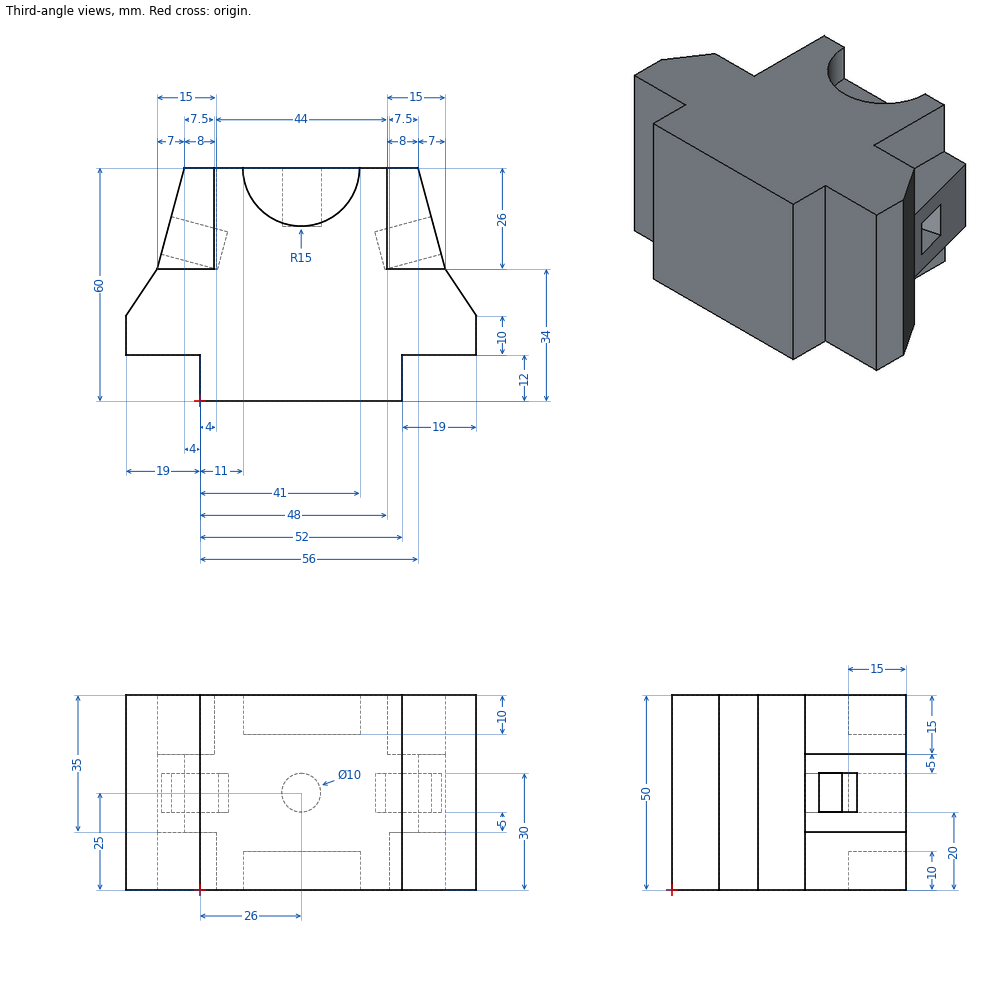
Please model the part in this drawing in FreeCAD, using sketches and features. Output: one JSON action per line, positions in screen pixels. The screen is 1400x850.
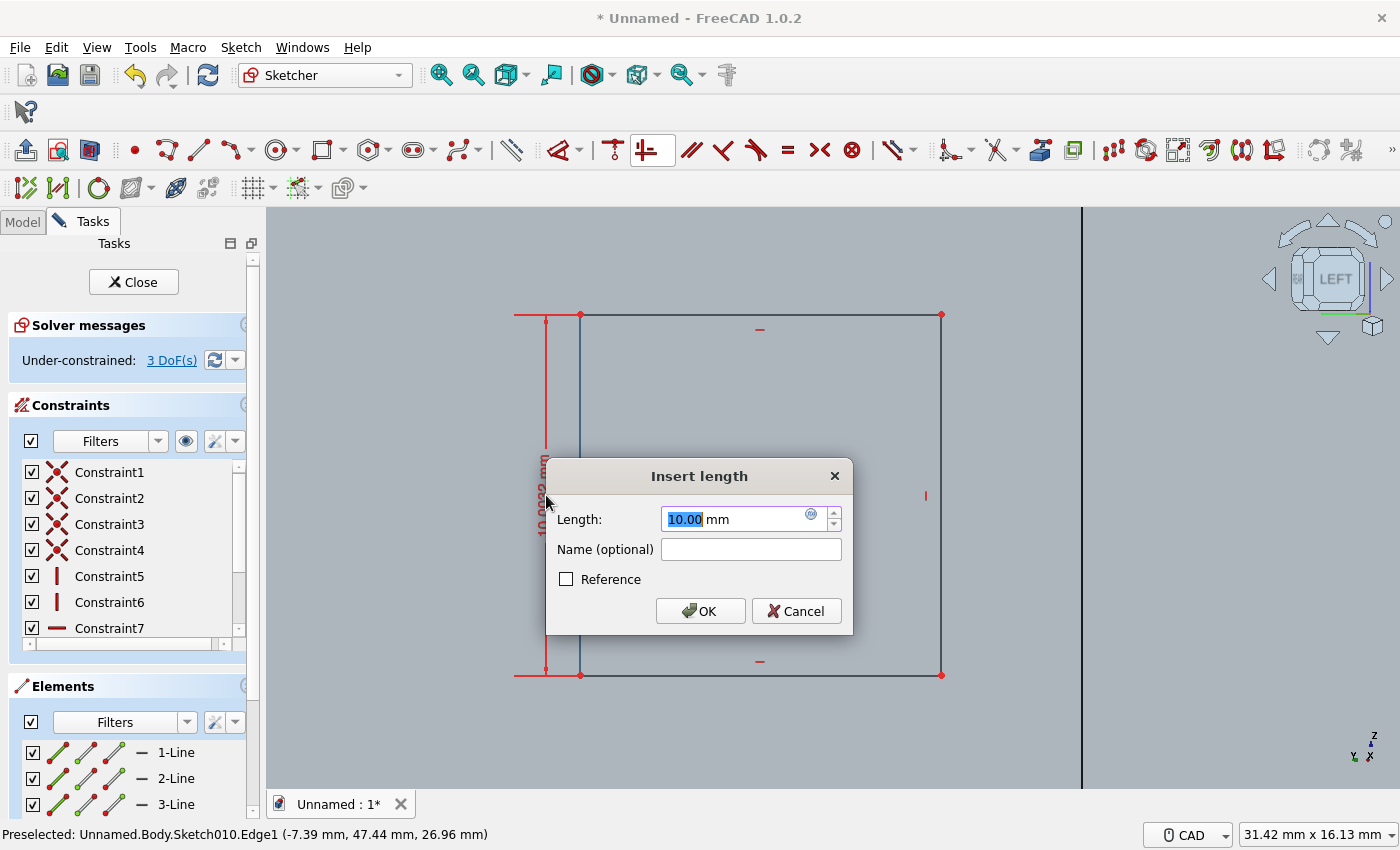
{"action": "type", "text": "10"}
{"action": "key", "text": "Return"}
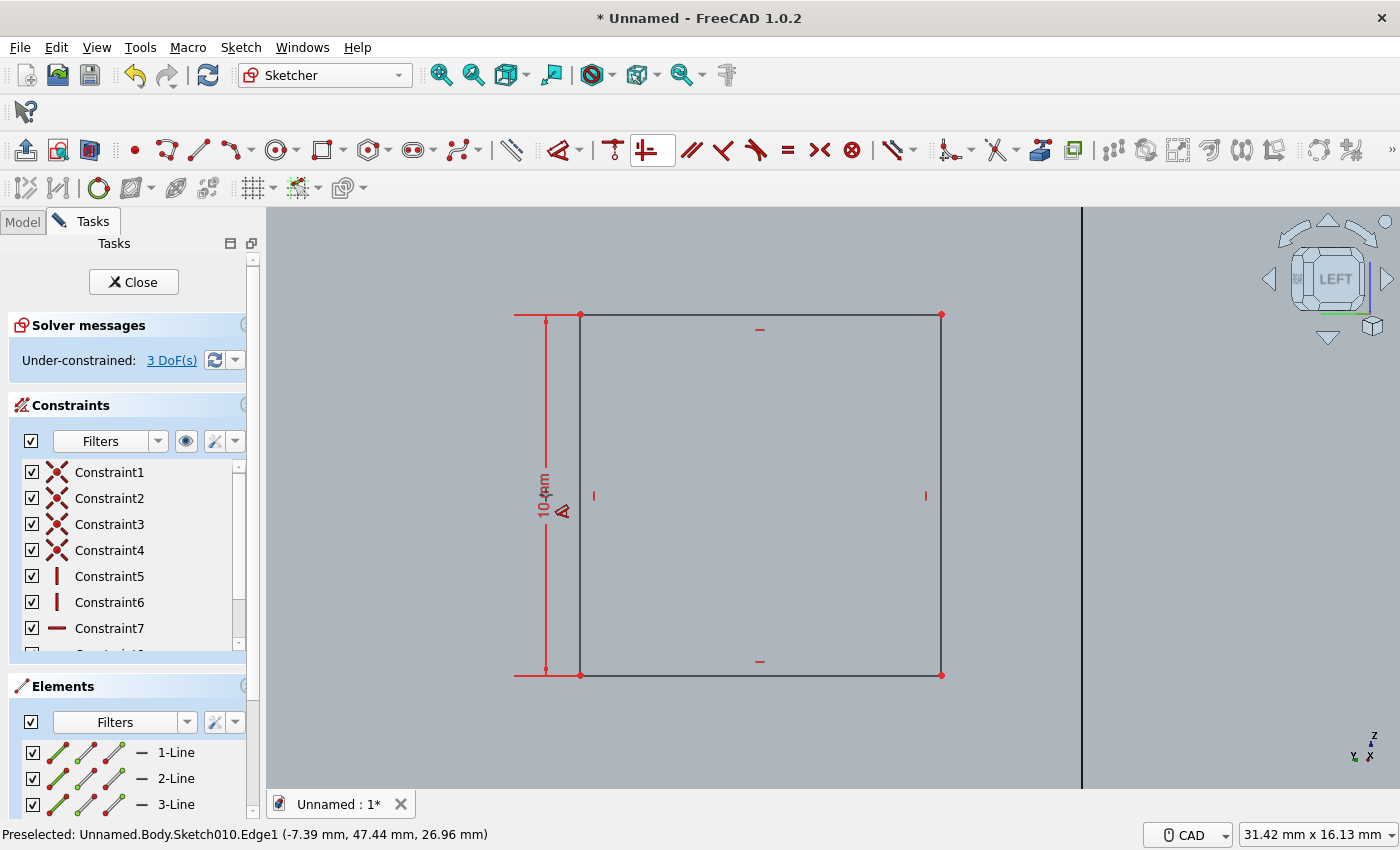
{"action": "left_click", "coordinate": [688, 676]}
{"action": "left_click", "coordinate": [760, 710]}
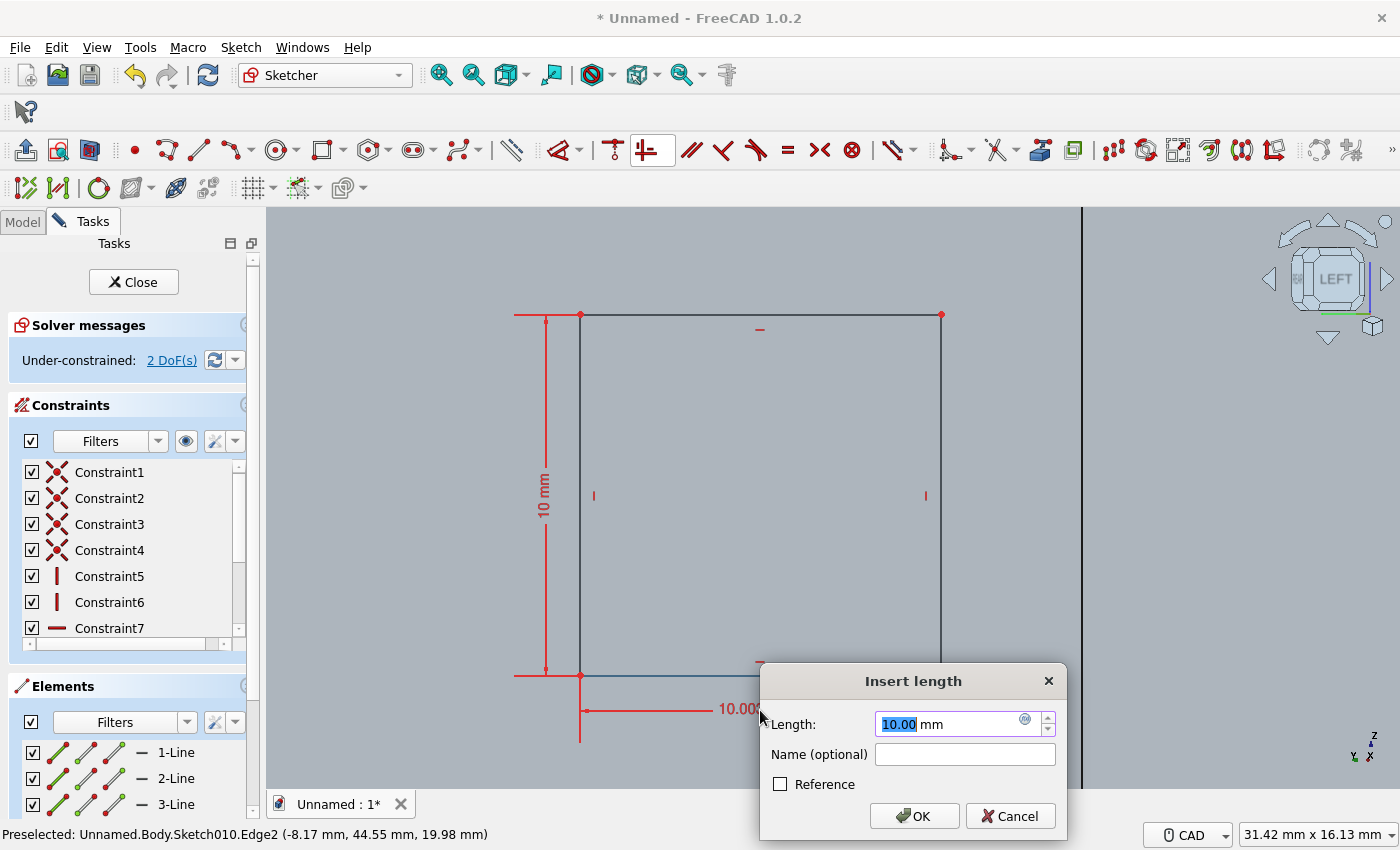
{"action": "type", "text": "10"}
{"action": "key", "text": "Return"}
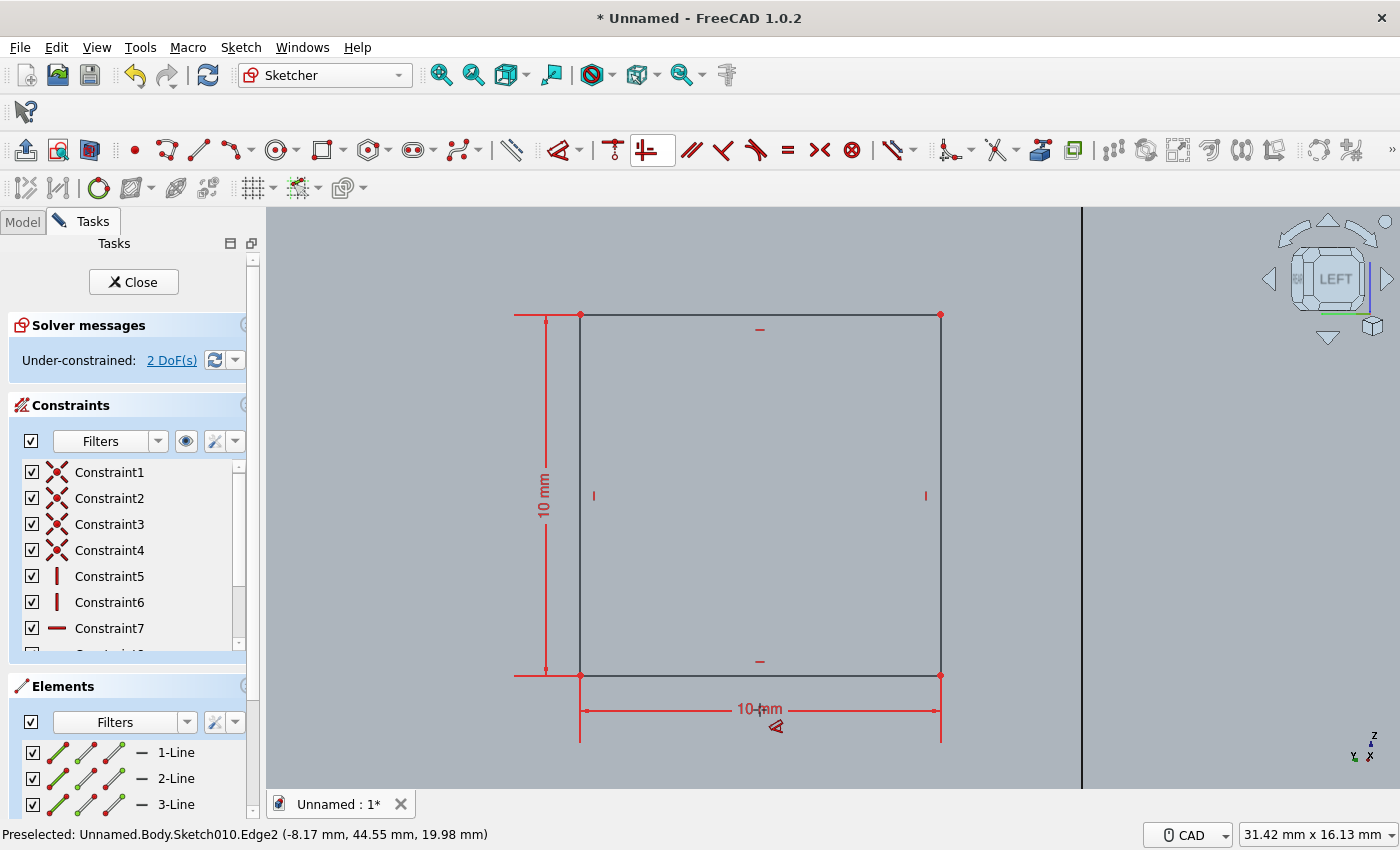
{"action": "left_click", "coordinate": [580, 315]}
{"action": "left_click", "coordinate": [546, 538]}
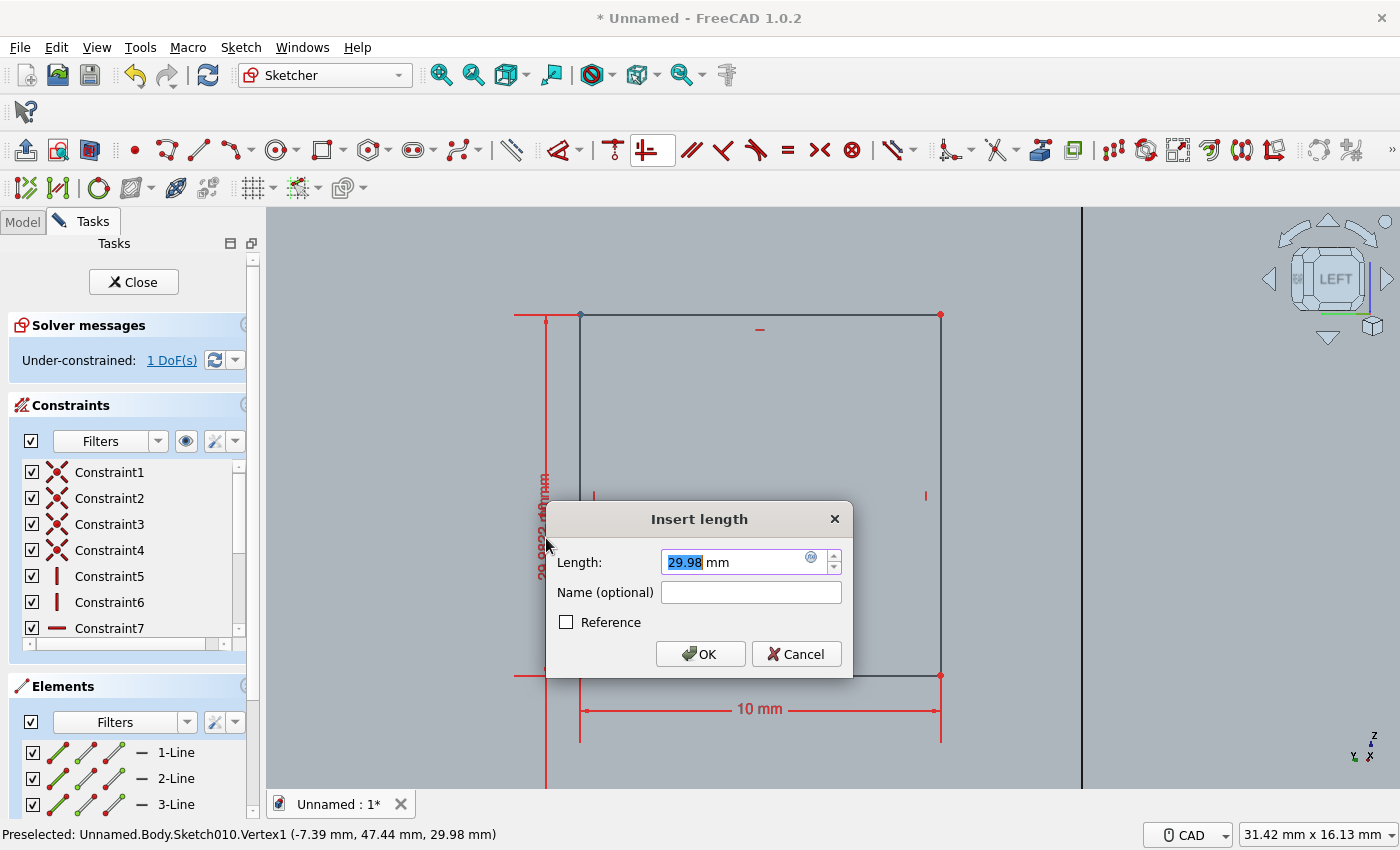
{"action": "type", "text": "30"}
{"action": "key", "text": "Return"}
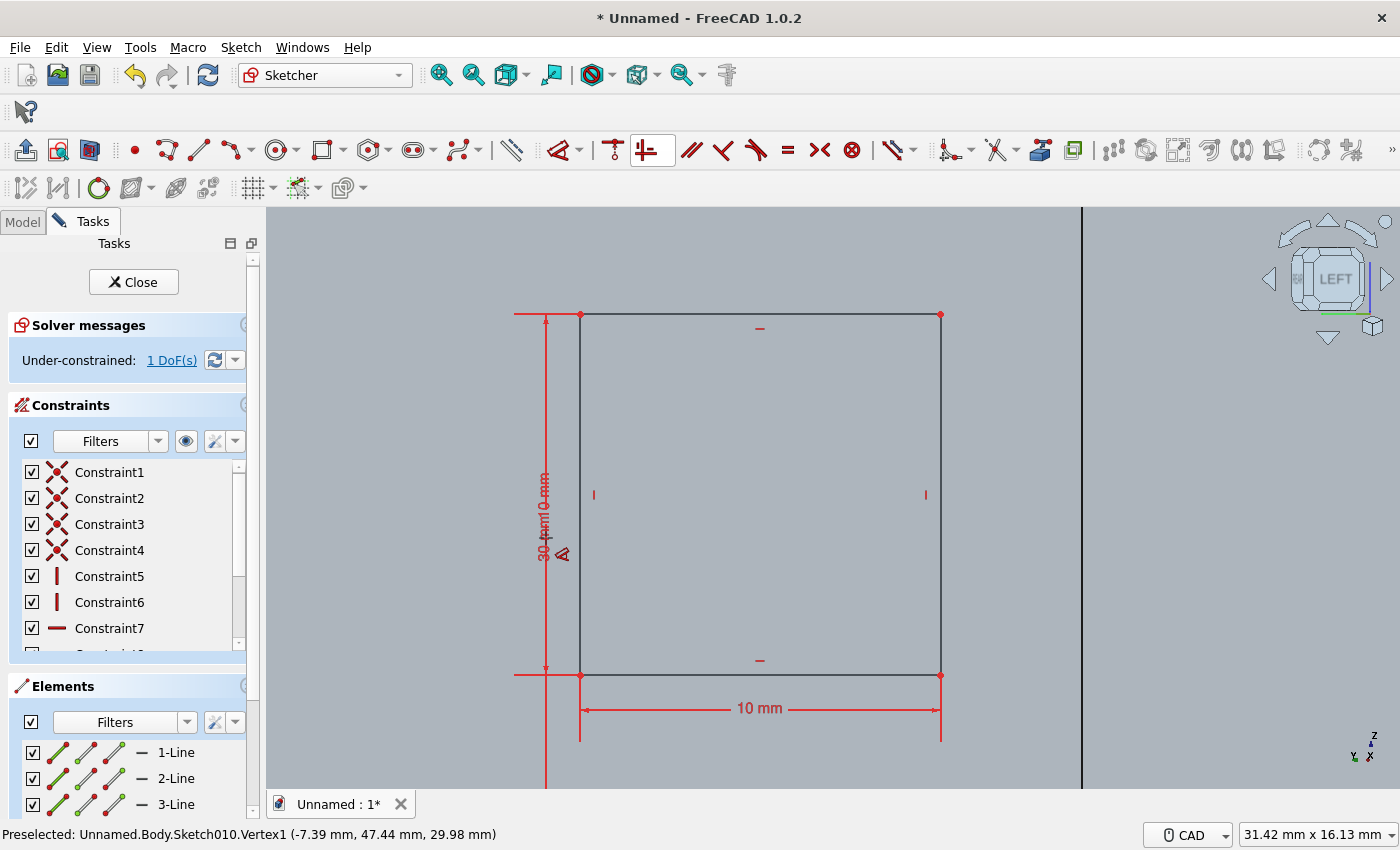
{"action": "left_click", "coordinate": [580, 314]}
{"action": "left_click", "coordinate": [907, 280]}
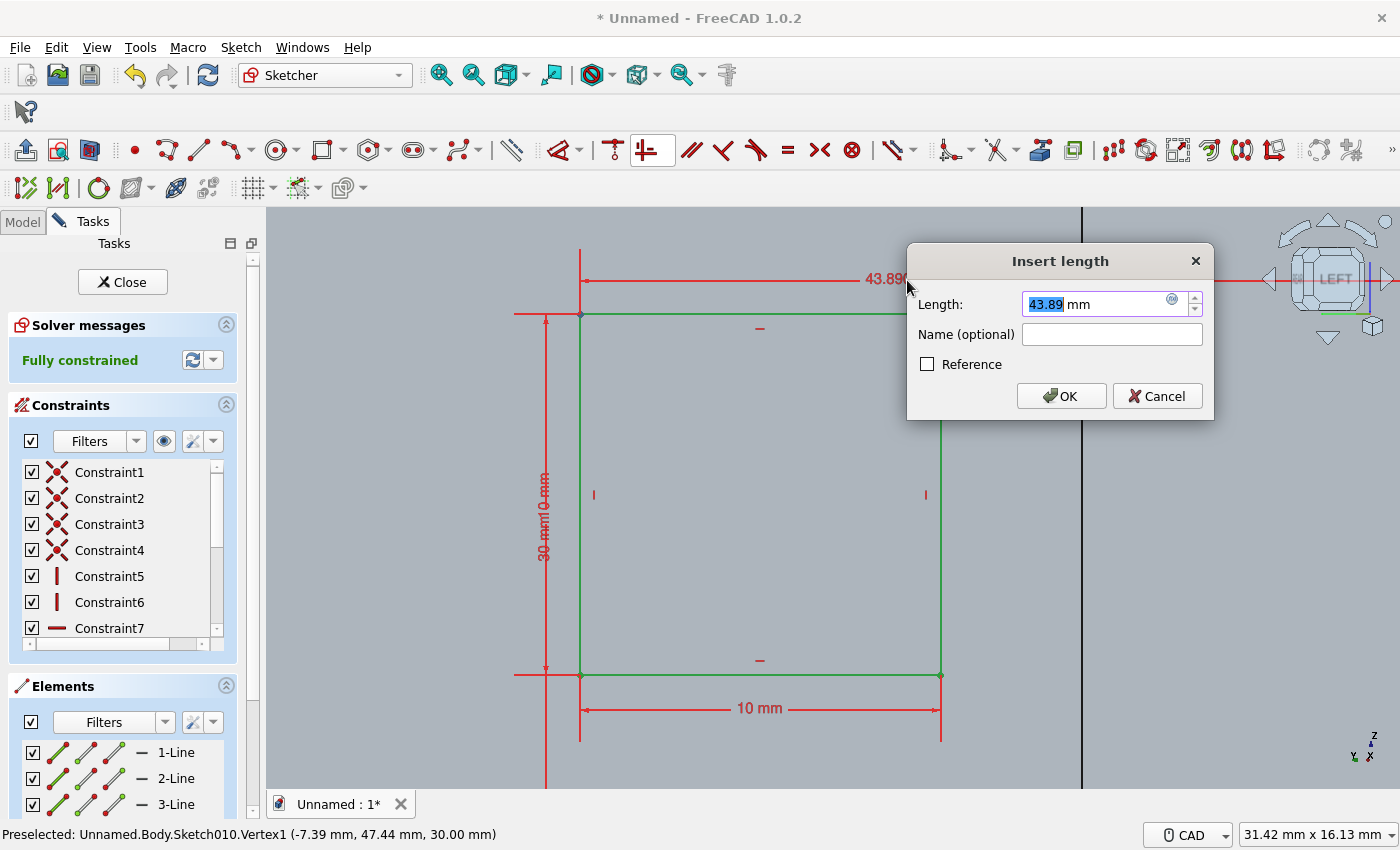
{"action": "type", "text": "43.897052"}
{"action": "key", "text": "Return"}
{"action": "key", "text": "Escape"}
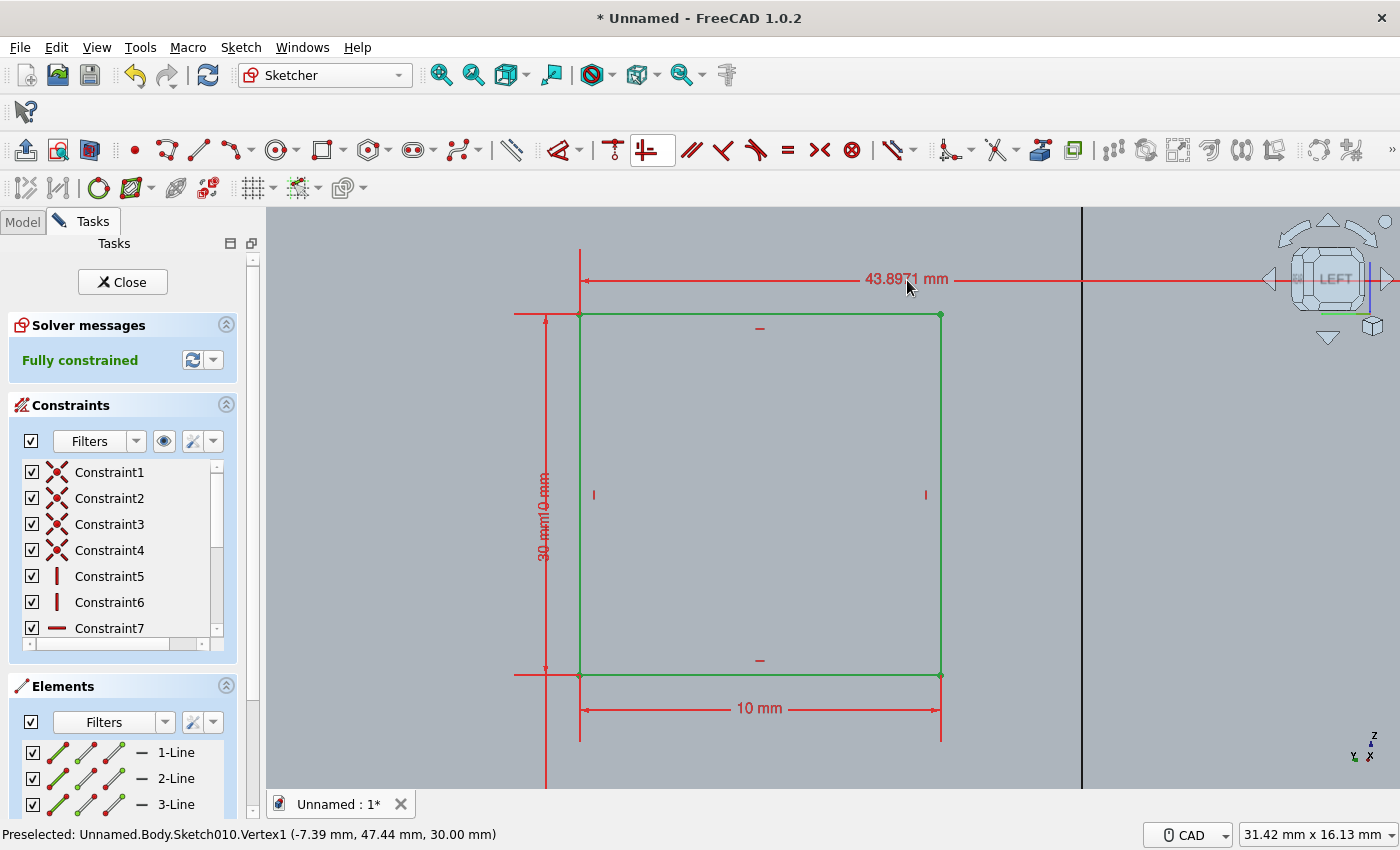
{"action": "left_click", "coordinate": [123, 282]}